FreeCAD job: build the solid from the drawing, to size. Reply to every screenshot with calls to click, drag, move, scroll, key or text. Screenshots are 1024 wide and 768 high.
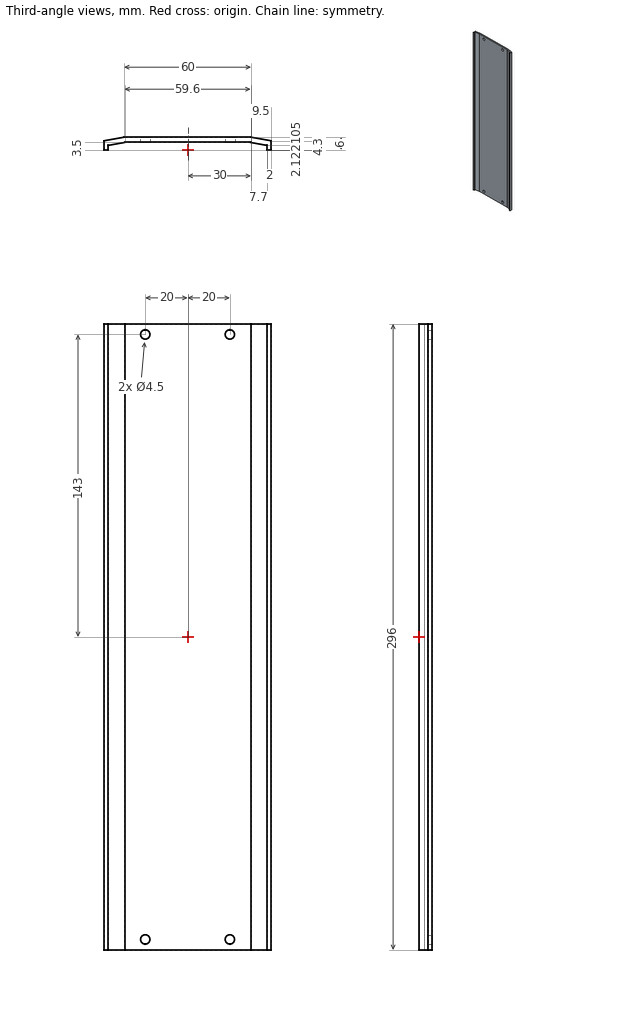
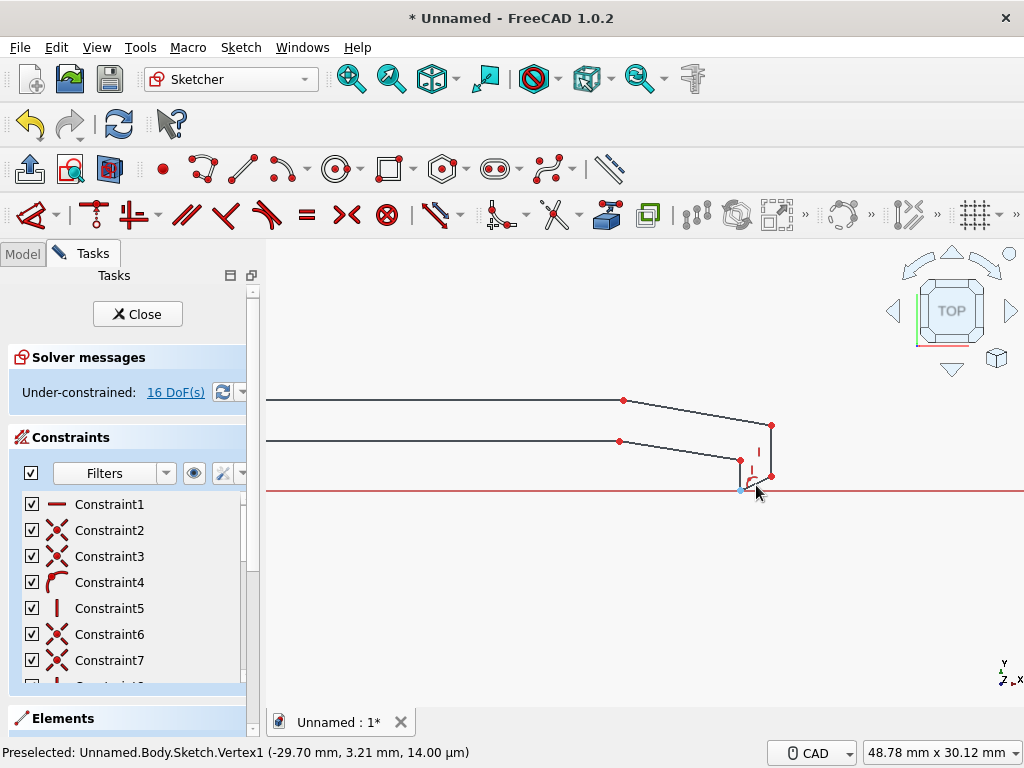
click(759, 482)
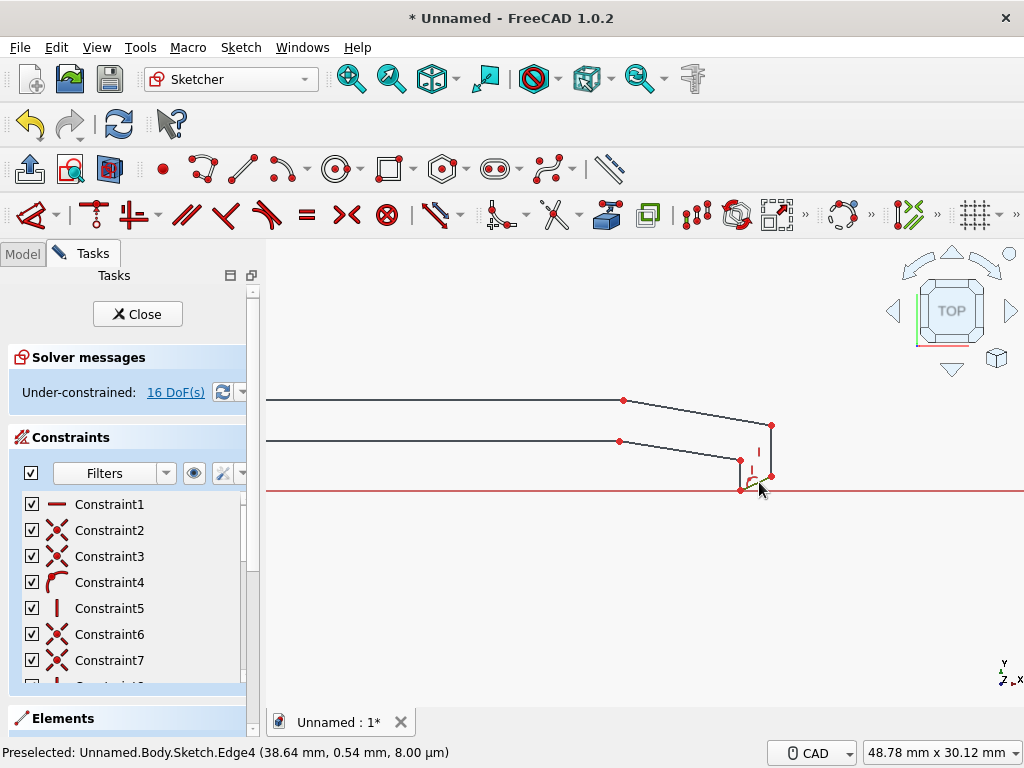
key(h)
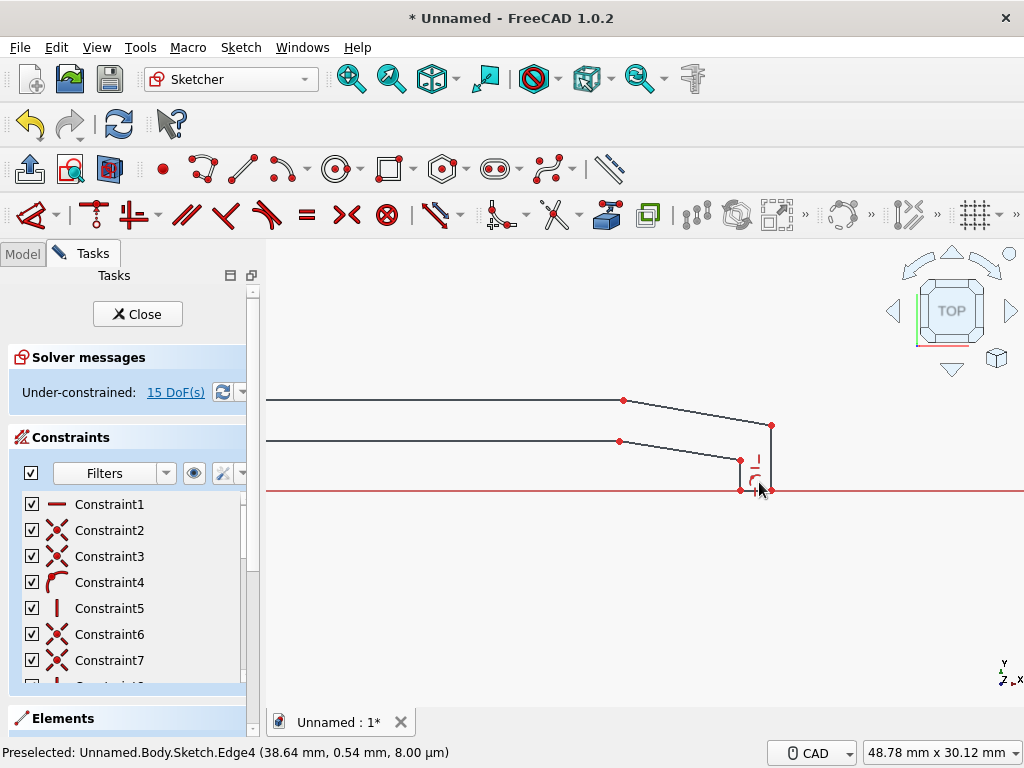
scroll(757, 485, down, 6)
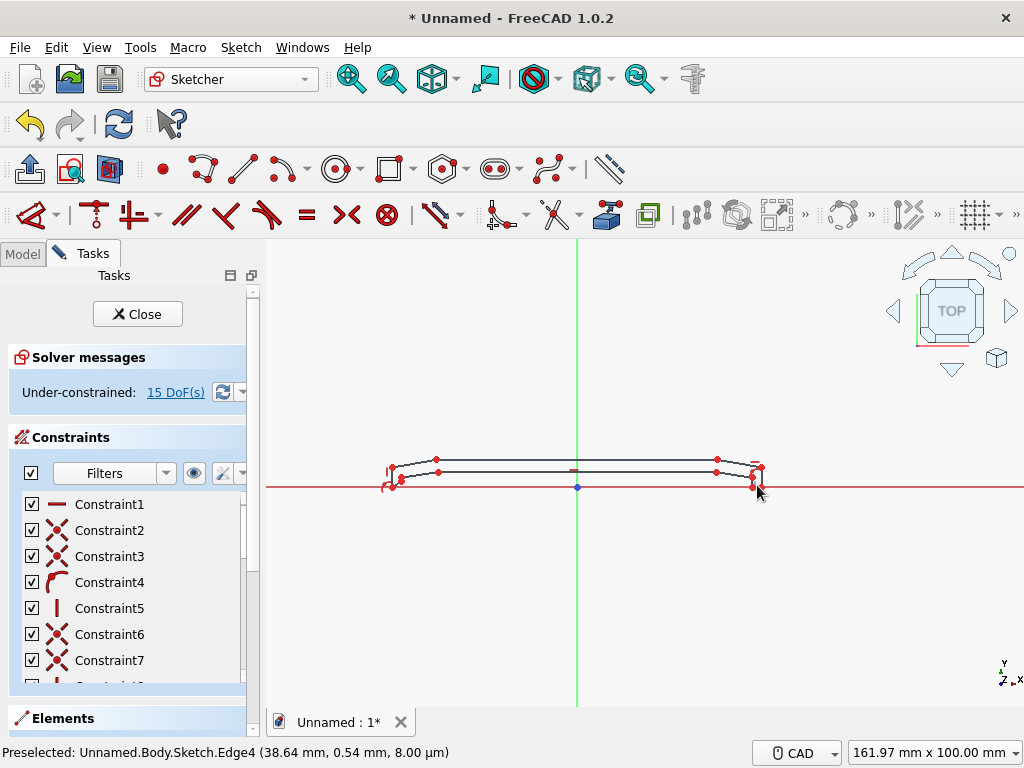
scroll(399, 483, up, 8)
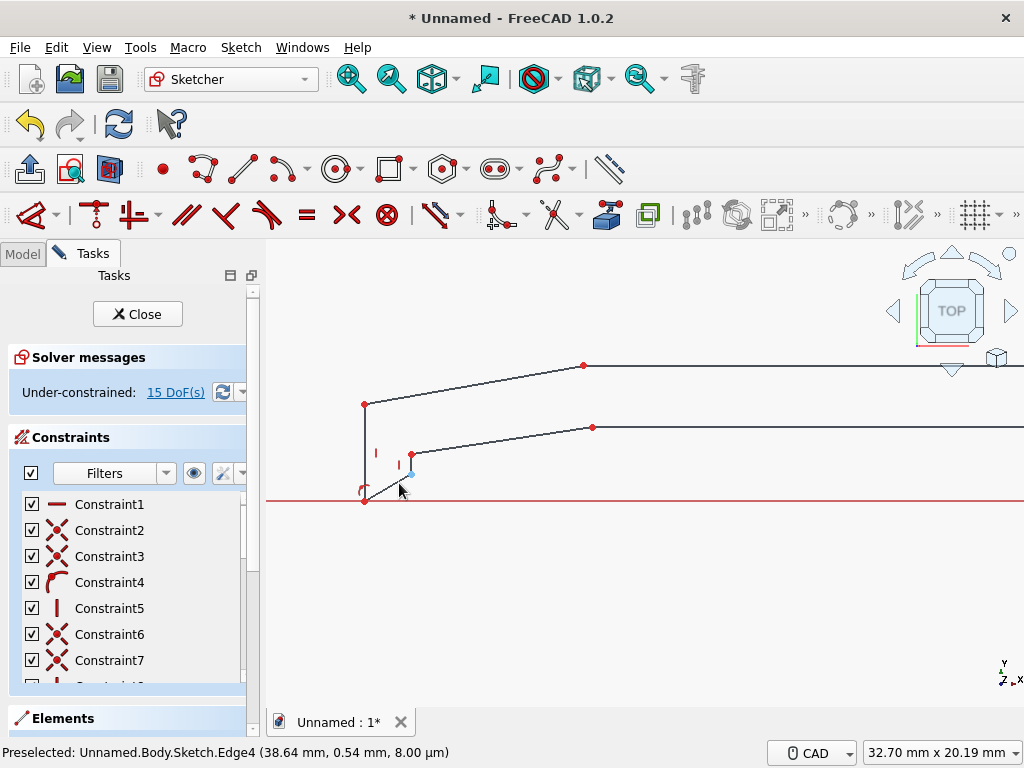
click(397, 482)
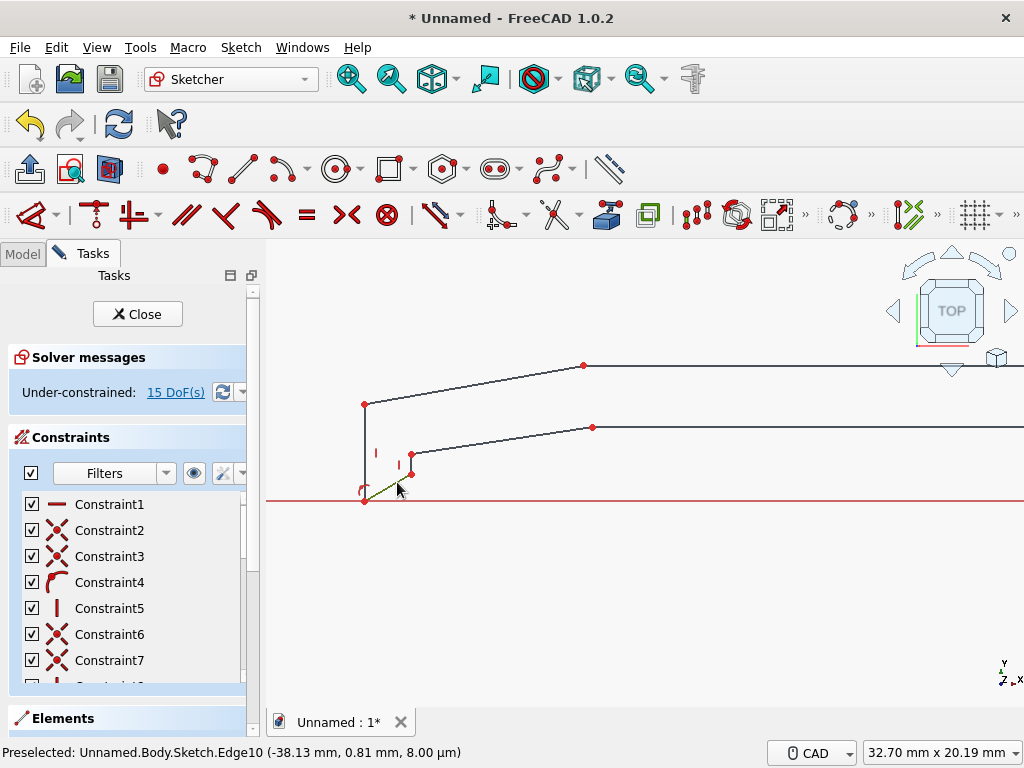
click(160, 216)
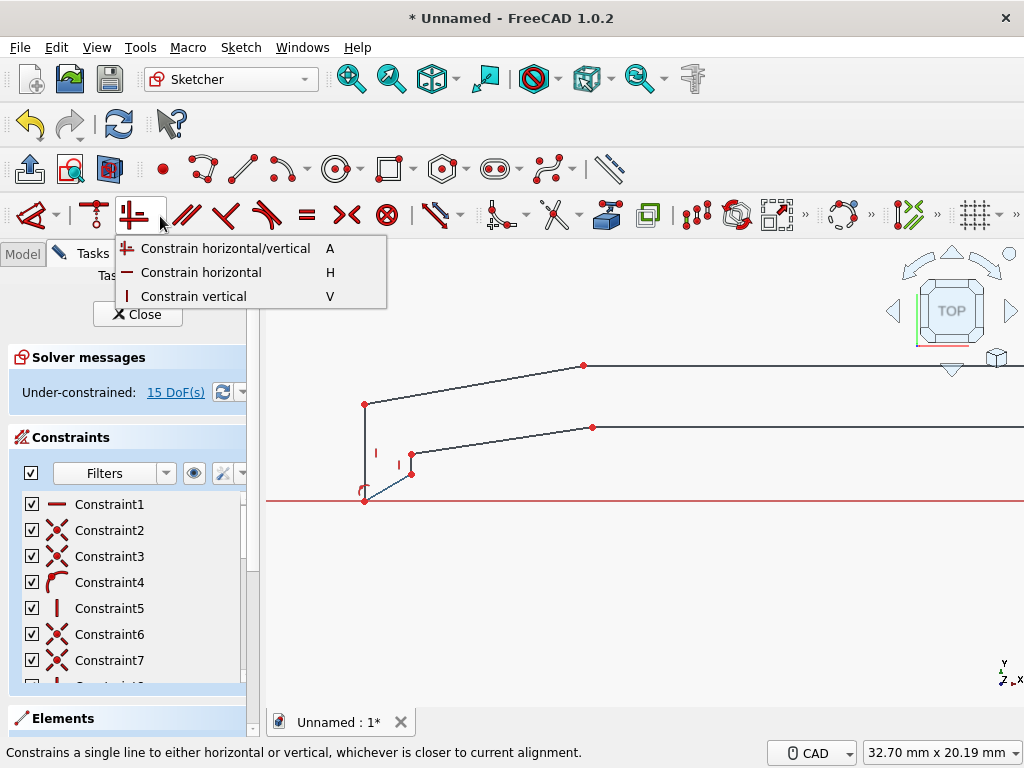
click(251, 272)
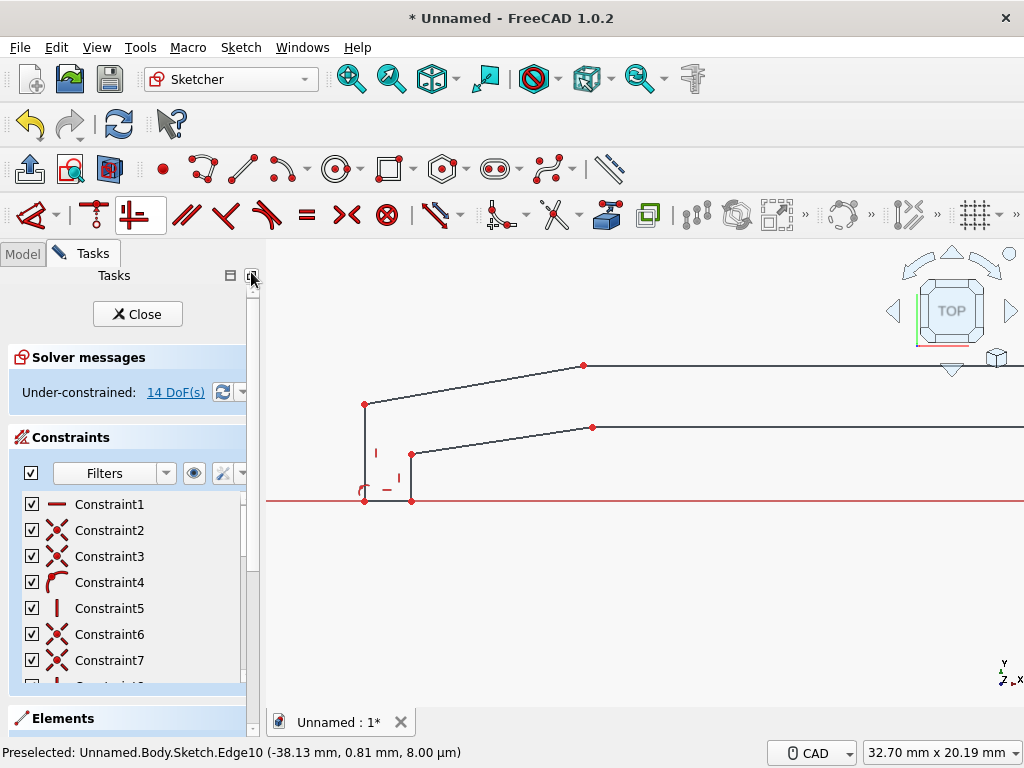
scroll(398, 483, down, 8)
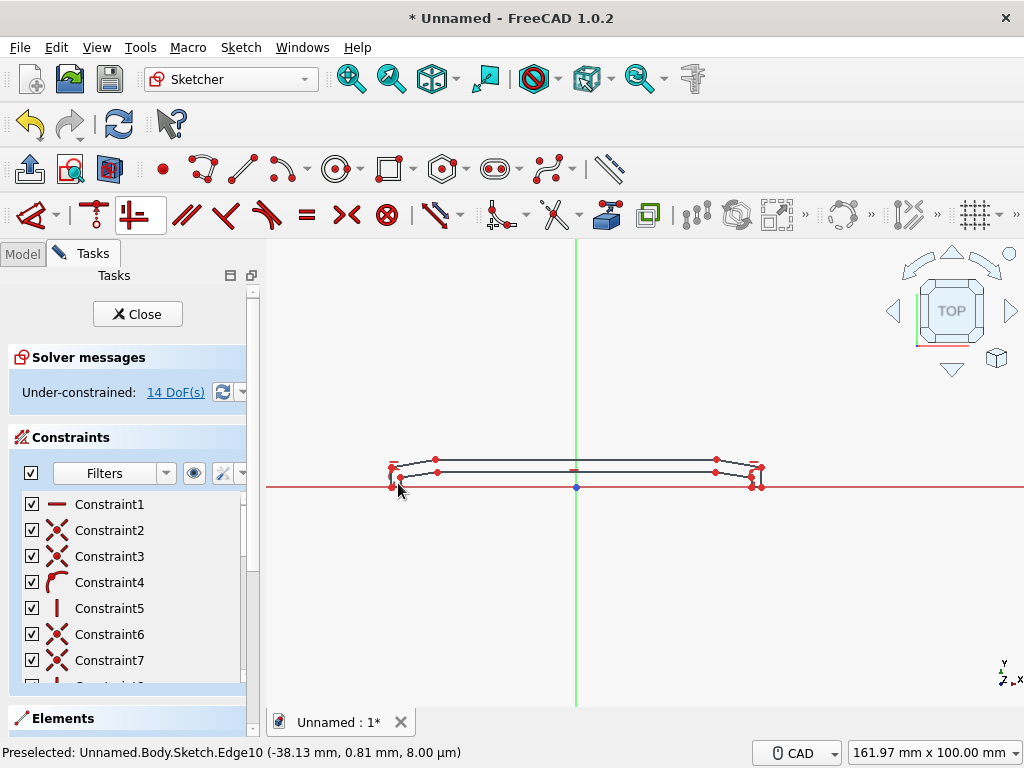
click(761, 467)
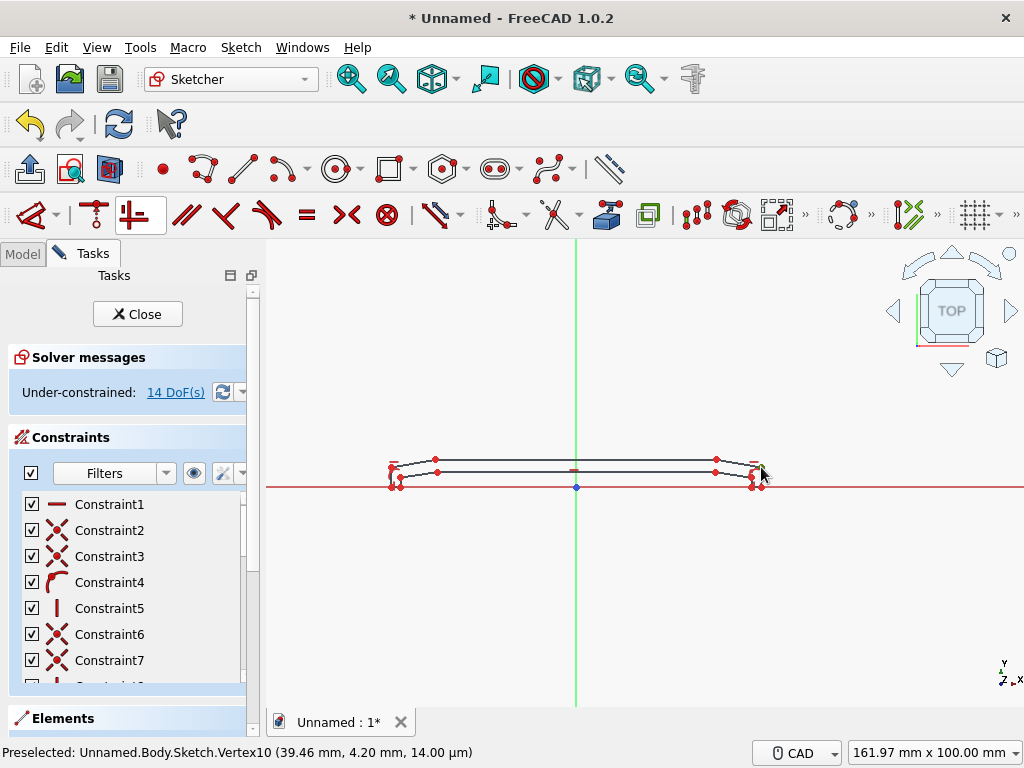
click(391, 468)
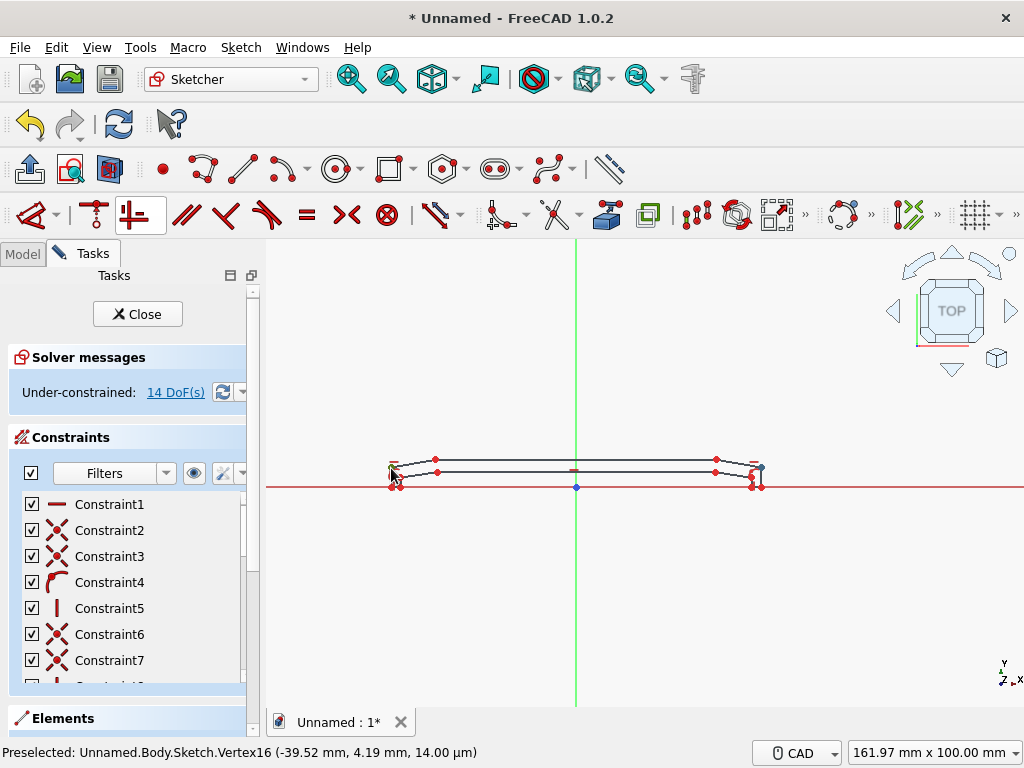
click(576, 650)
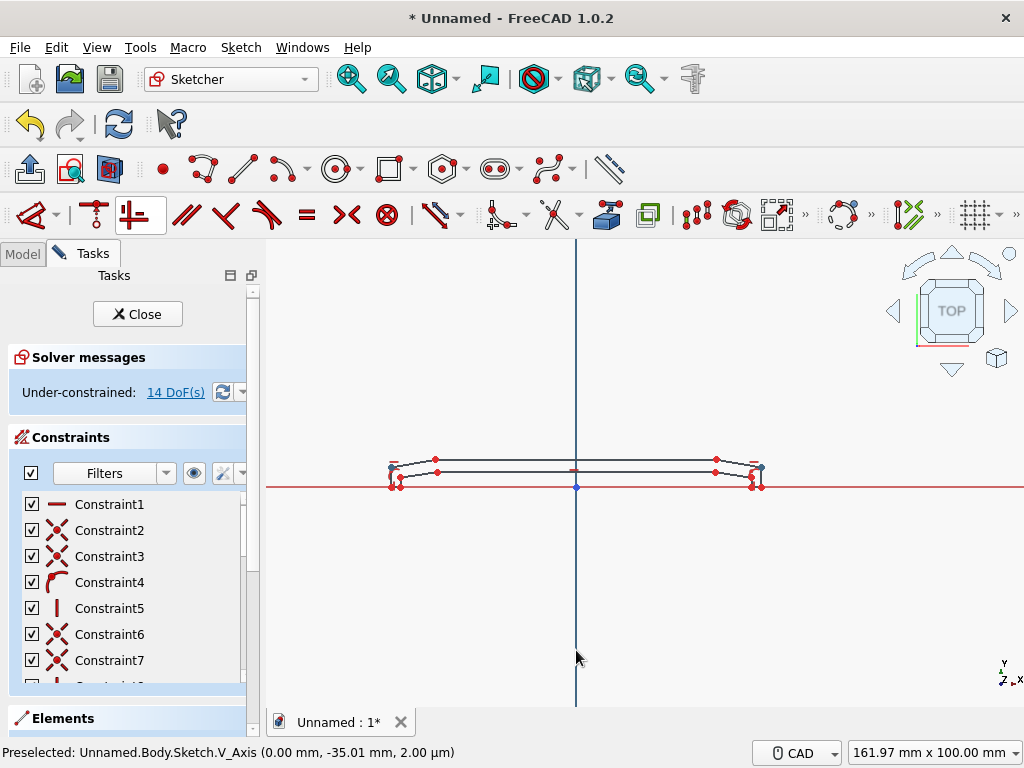
click(348, 216)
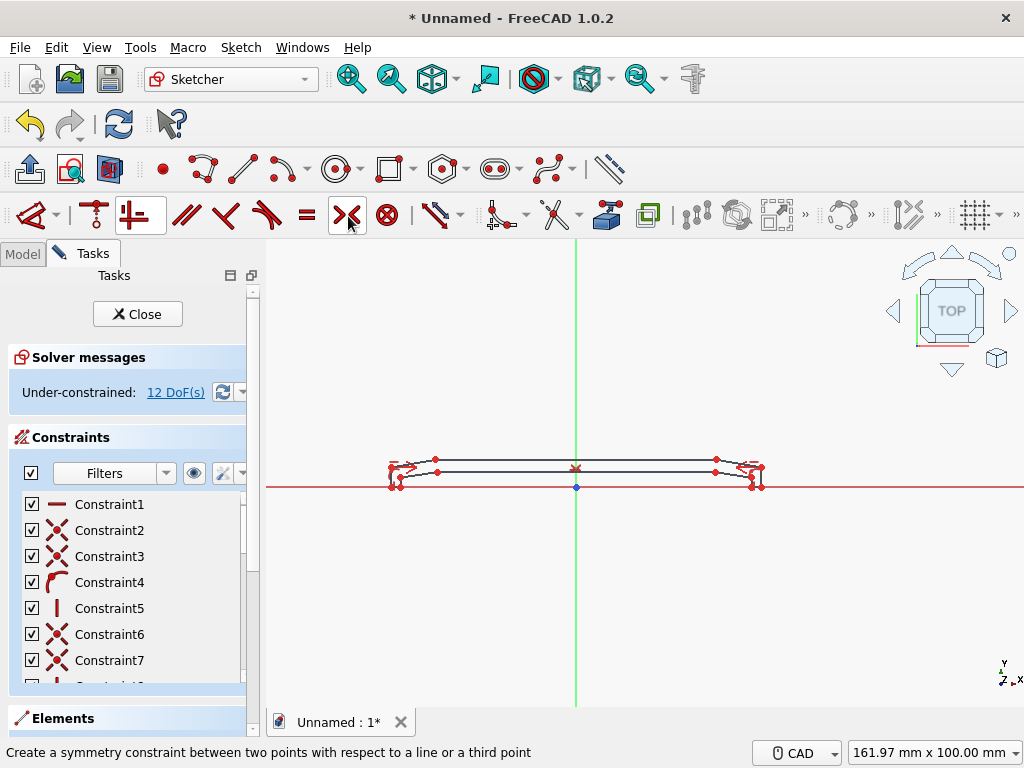
scroll(752, 478, up, 2)